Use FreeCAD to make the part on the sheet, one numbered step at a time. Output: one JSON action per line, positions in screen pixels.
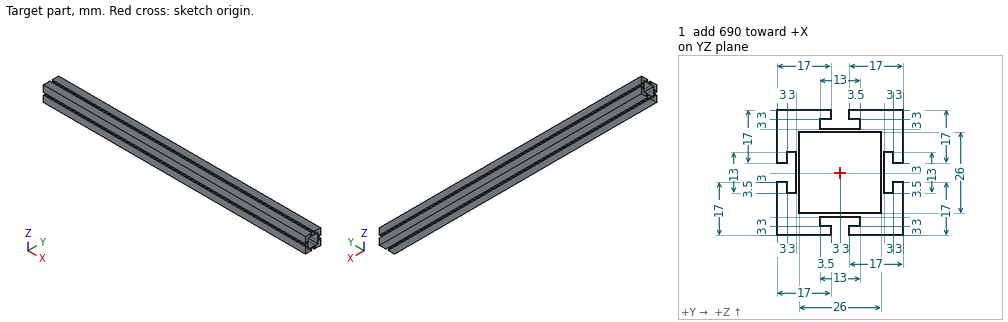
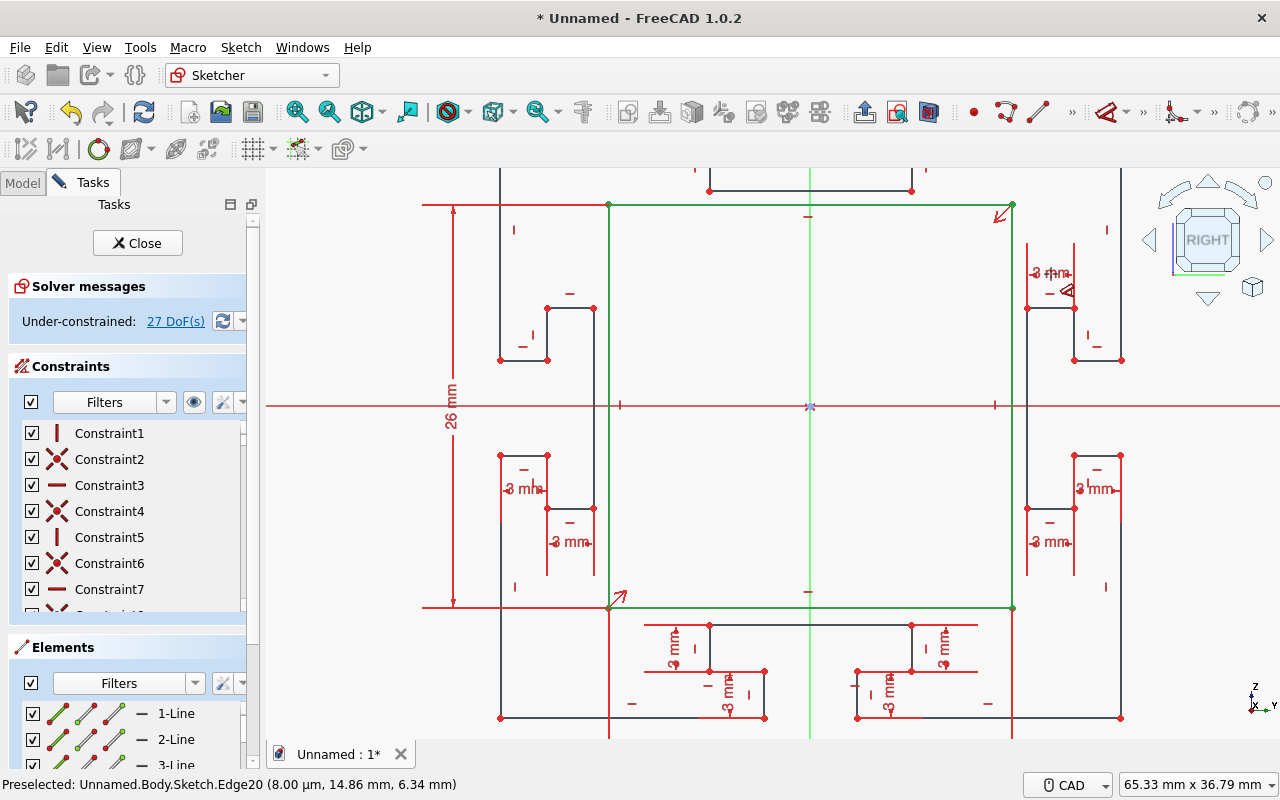
{"action": "left_click", "coordinate": [1088, 361]}
{"action": "left_click", "coordinate": [1095, 327]}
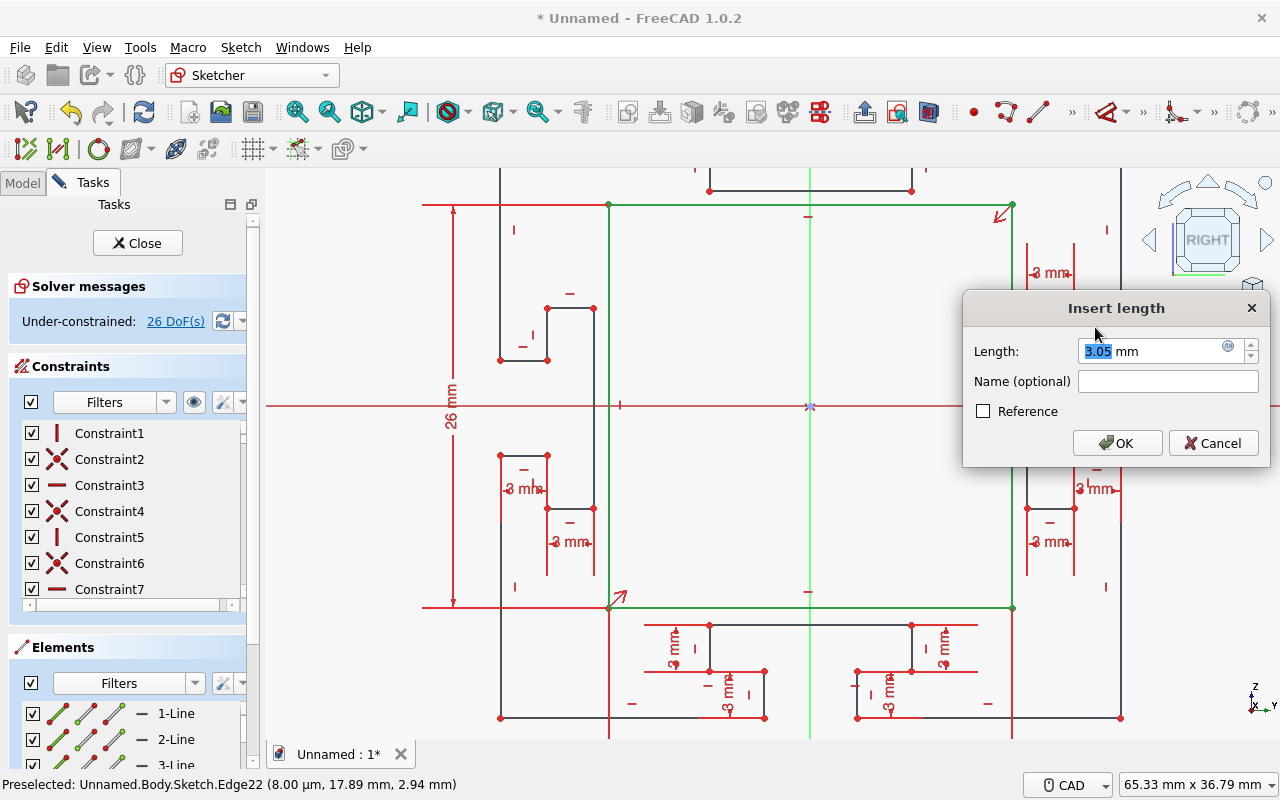
{"action": "type", "text": "3"}
{"action": "key", "text": "Return"}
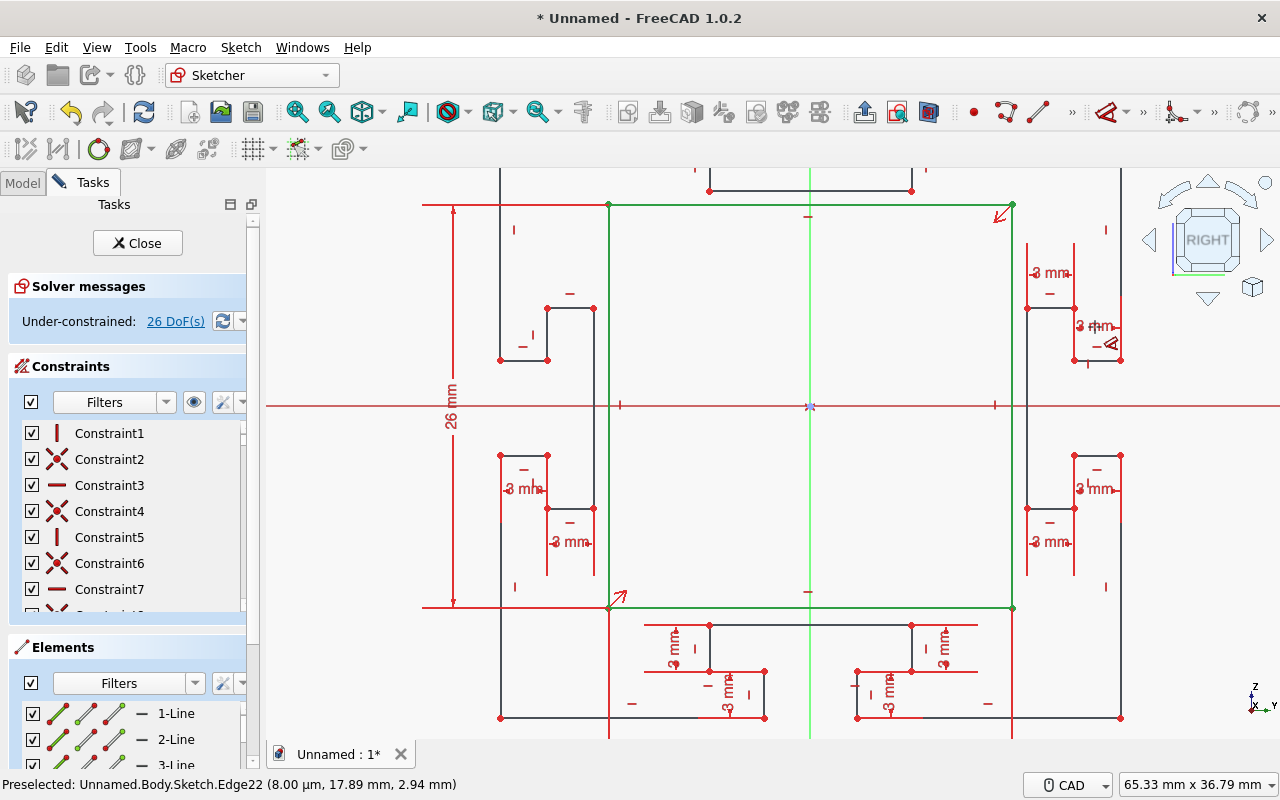
{"action": "scroll", "coordinate": [576, 511], "scroll_direction": "down", "scroll_amount": 3}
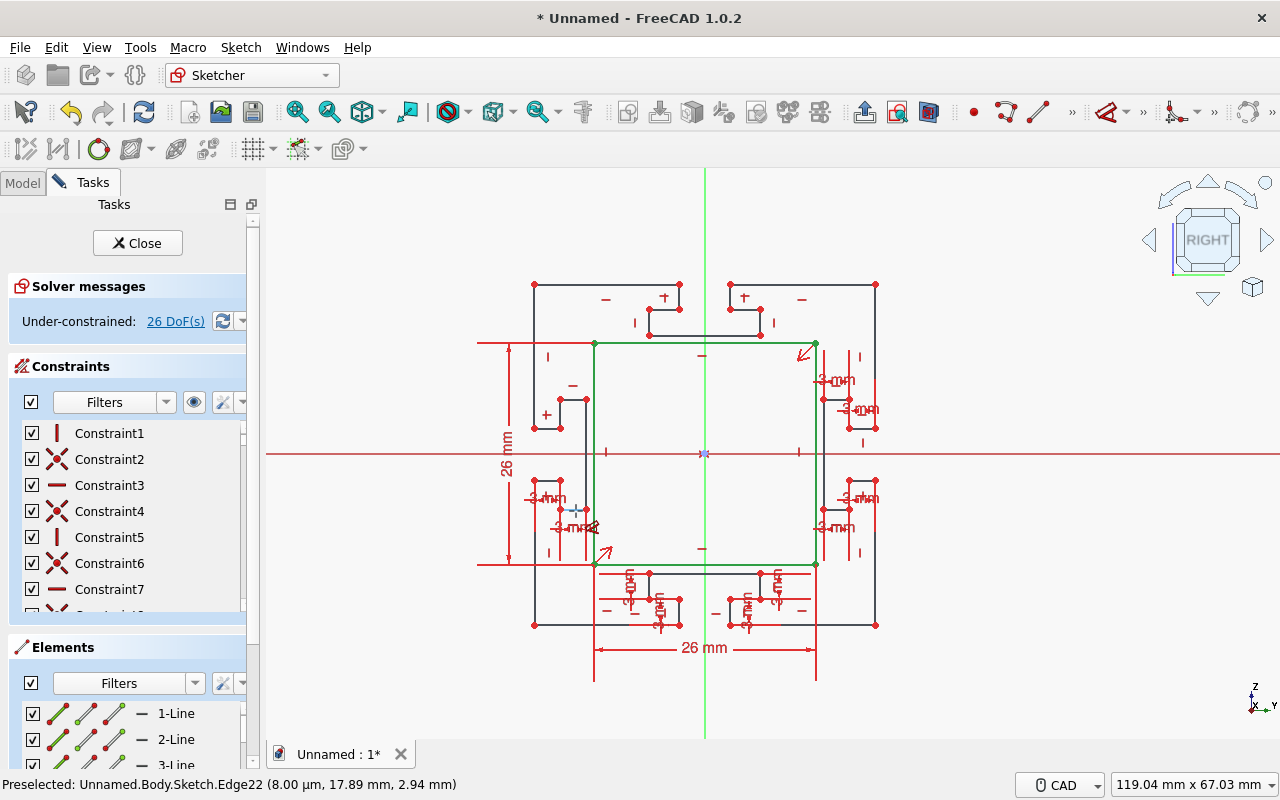
{"action": "scroll", "coordinate": [730, 292], "scroll_direction": "up", "scroll_amount": 4}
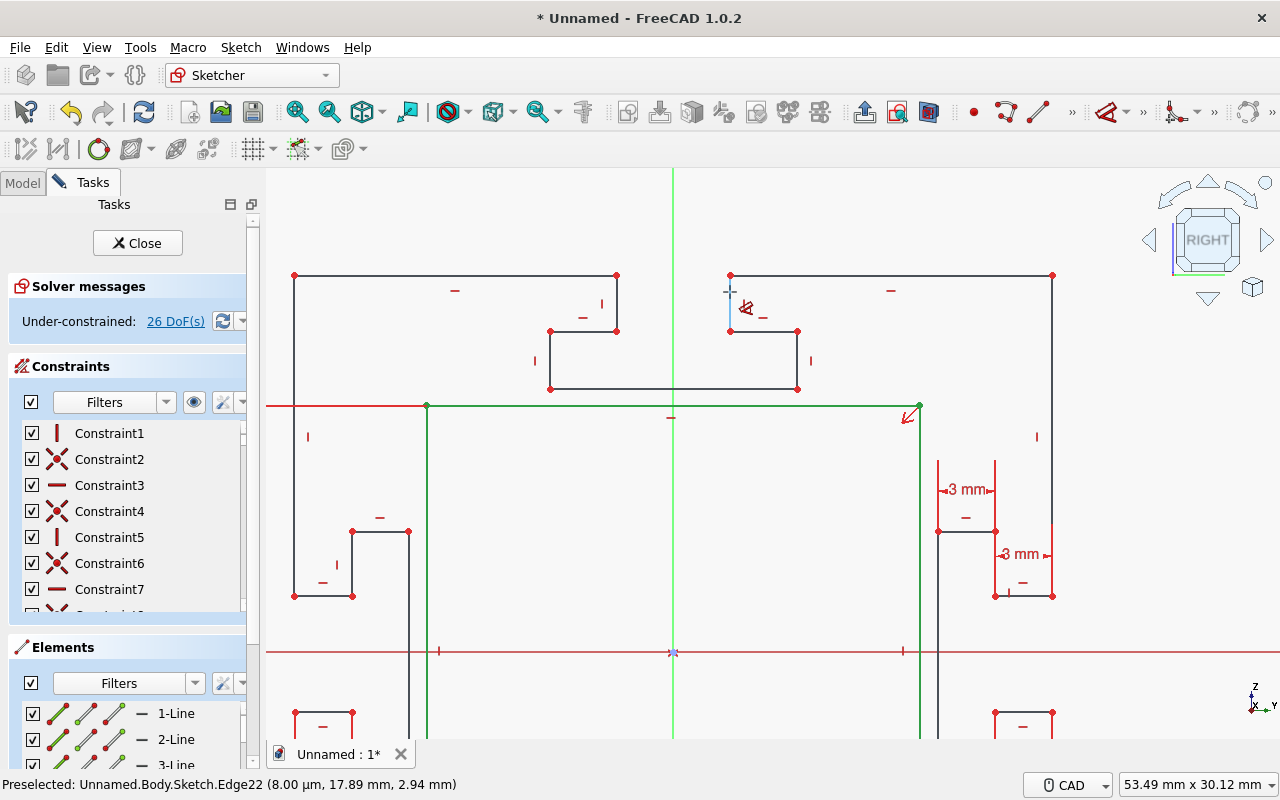
{"action": "left_click", "coordinate": [730, 293]}
{"action": "left_click", "coordinate": [764, 304]}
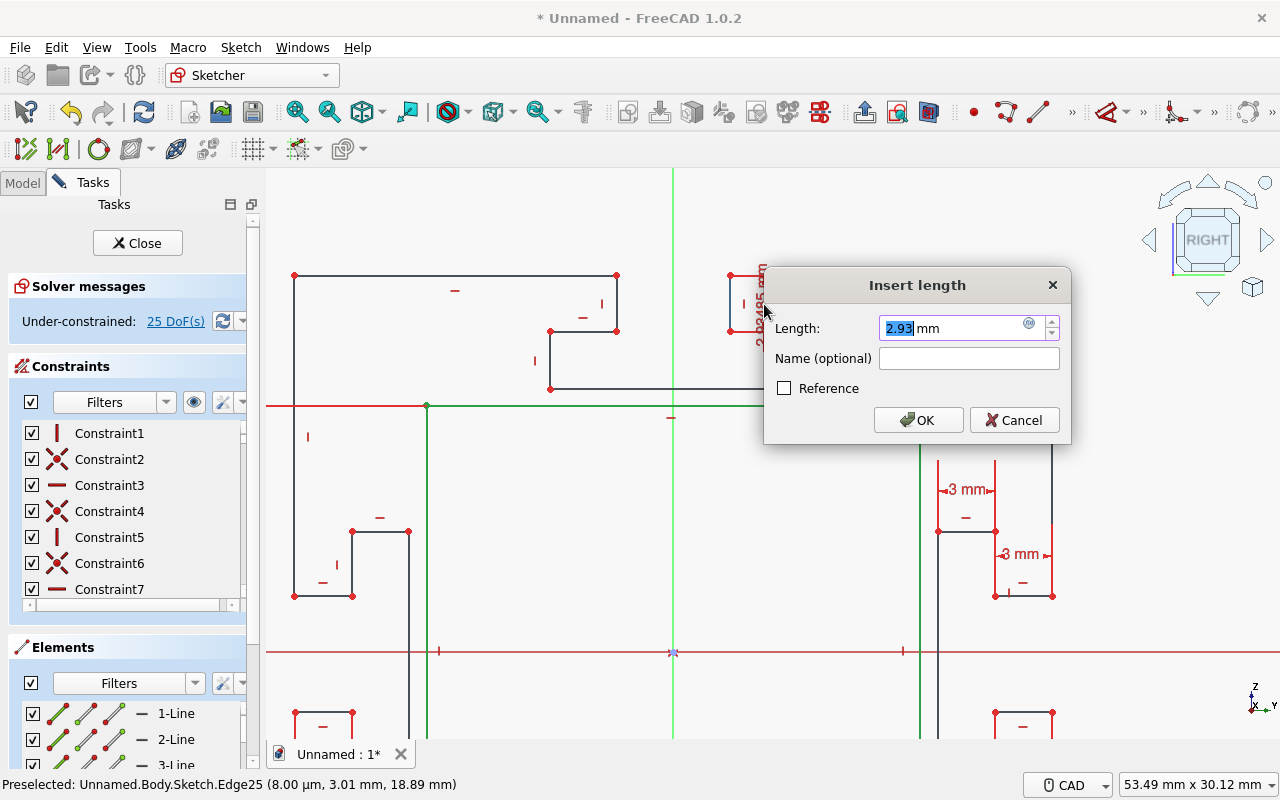
{"action": "type", "text": "3"}
{"action": "key", "text": "Return"}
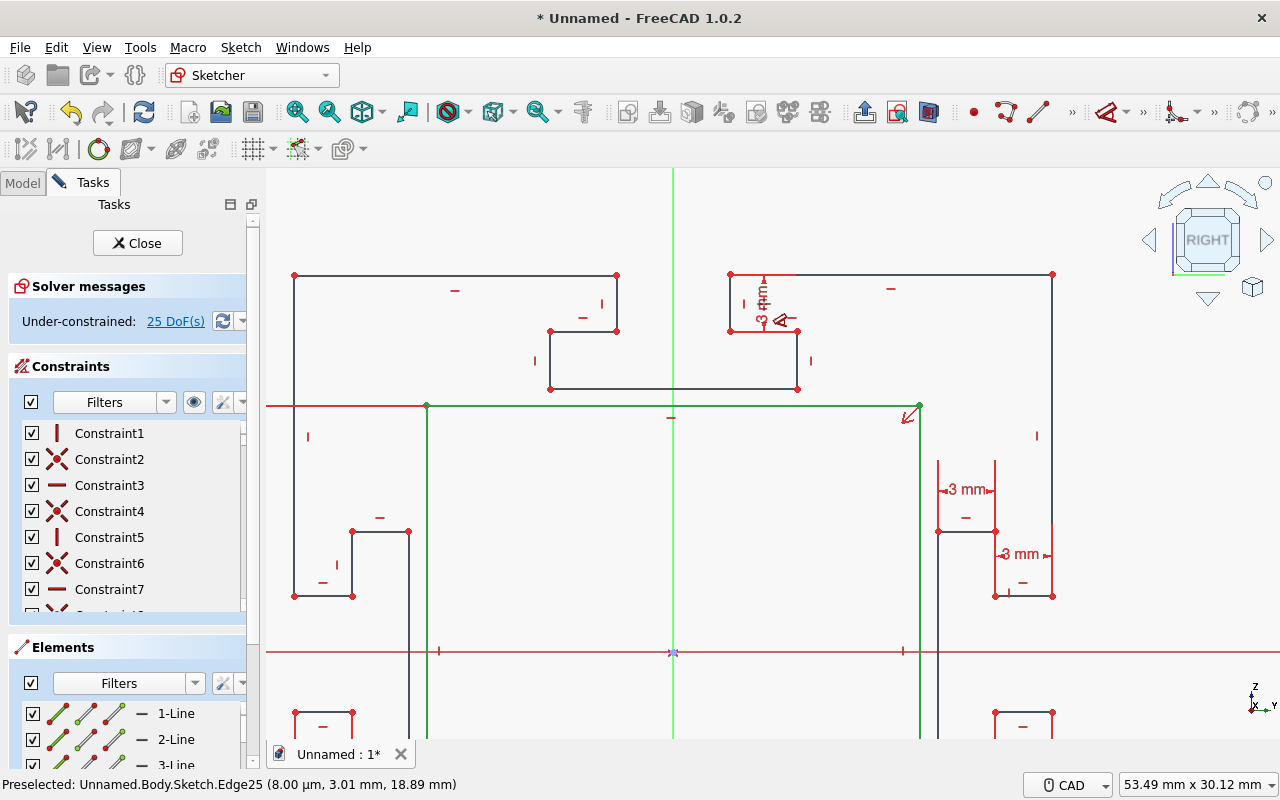
{"action": "left_click", "coordinate": [797, 349]}
{"action": "left_click", "coordinate": [831, 361]}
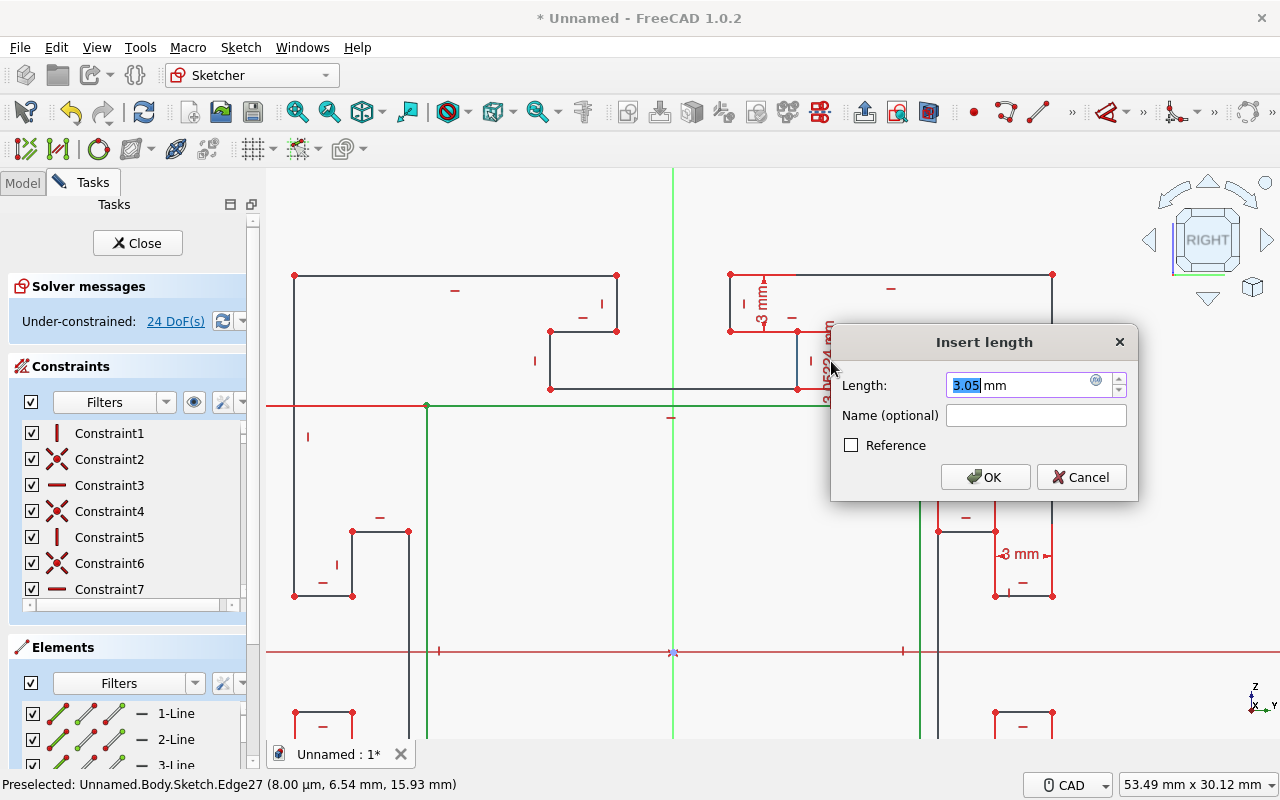
{"action": "type", "text": "3"}
{"action": "key", "text": "Return"}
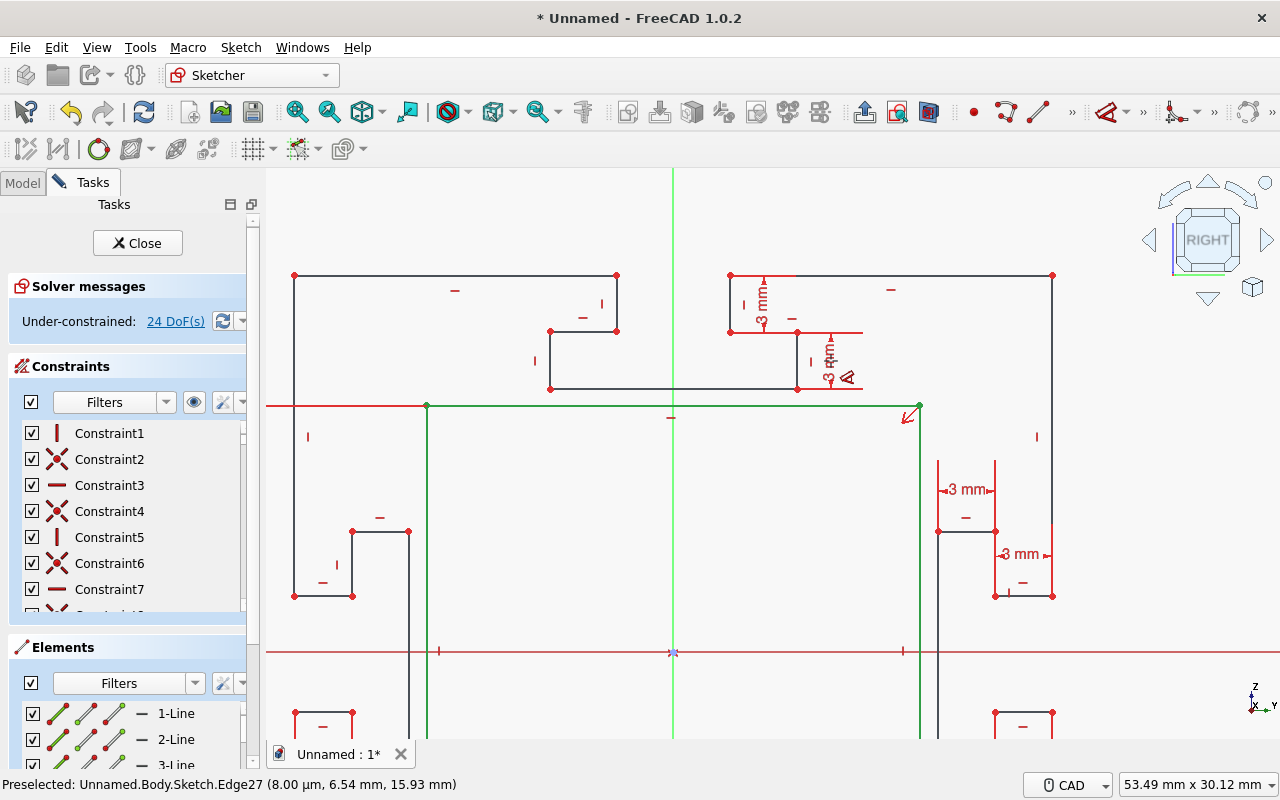
{"action": "left_click", "coordinate": [550, 372]}
{"action": "left_click", "coordinate": [516, 361]}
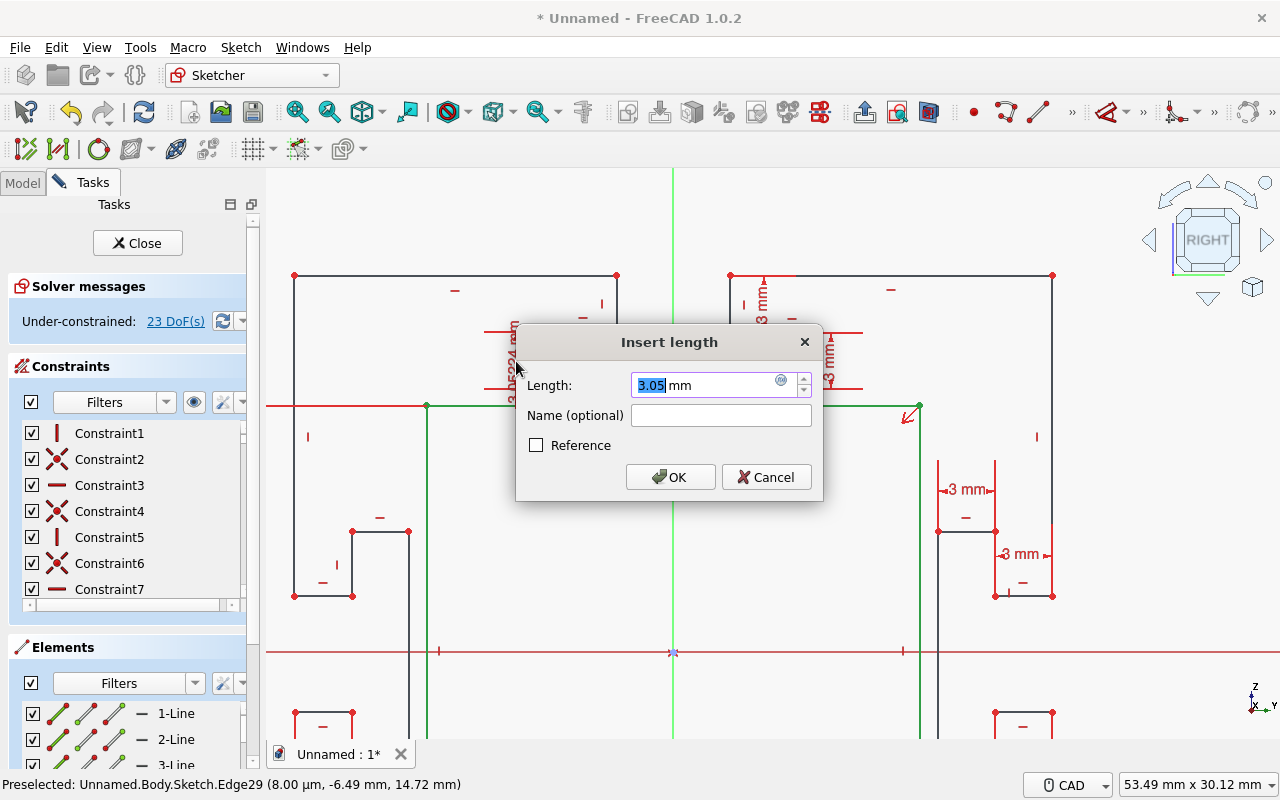
{"action": "type", "text": "3"}
{"action": "key", "text": "Return"}